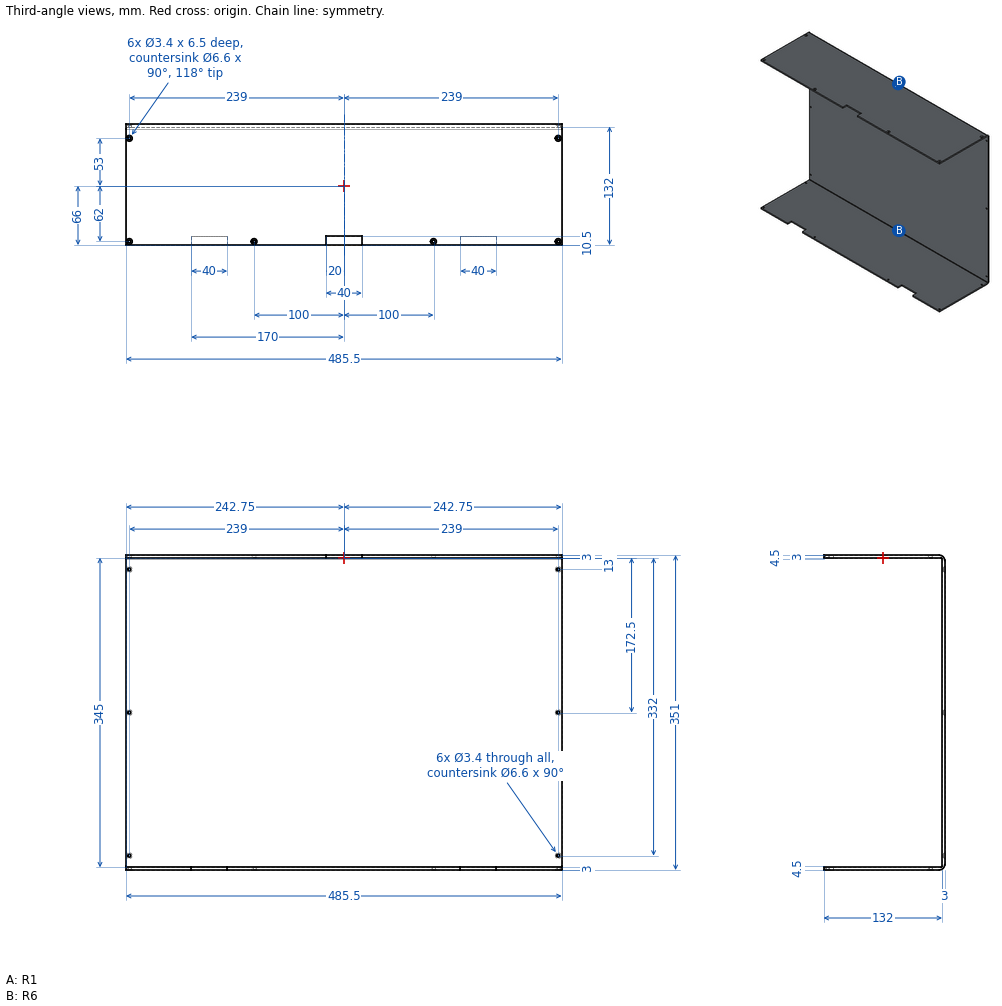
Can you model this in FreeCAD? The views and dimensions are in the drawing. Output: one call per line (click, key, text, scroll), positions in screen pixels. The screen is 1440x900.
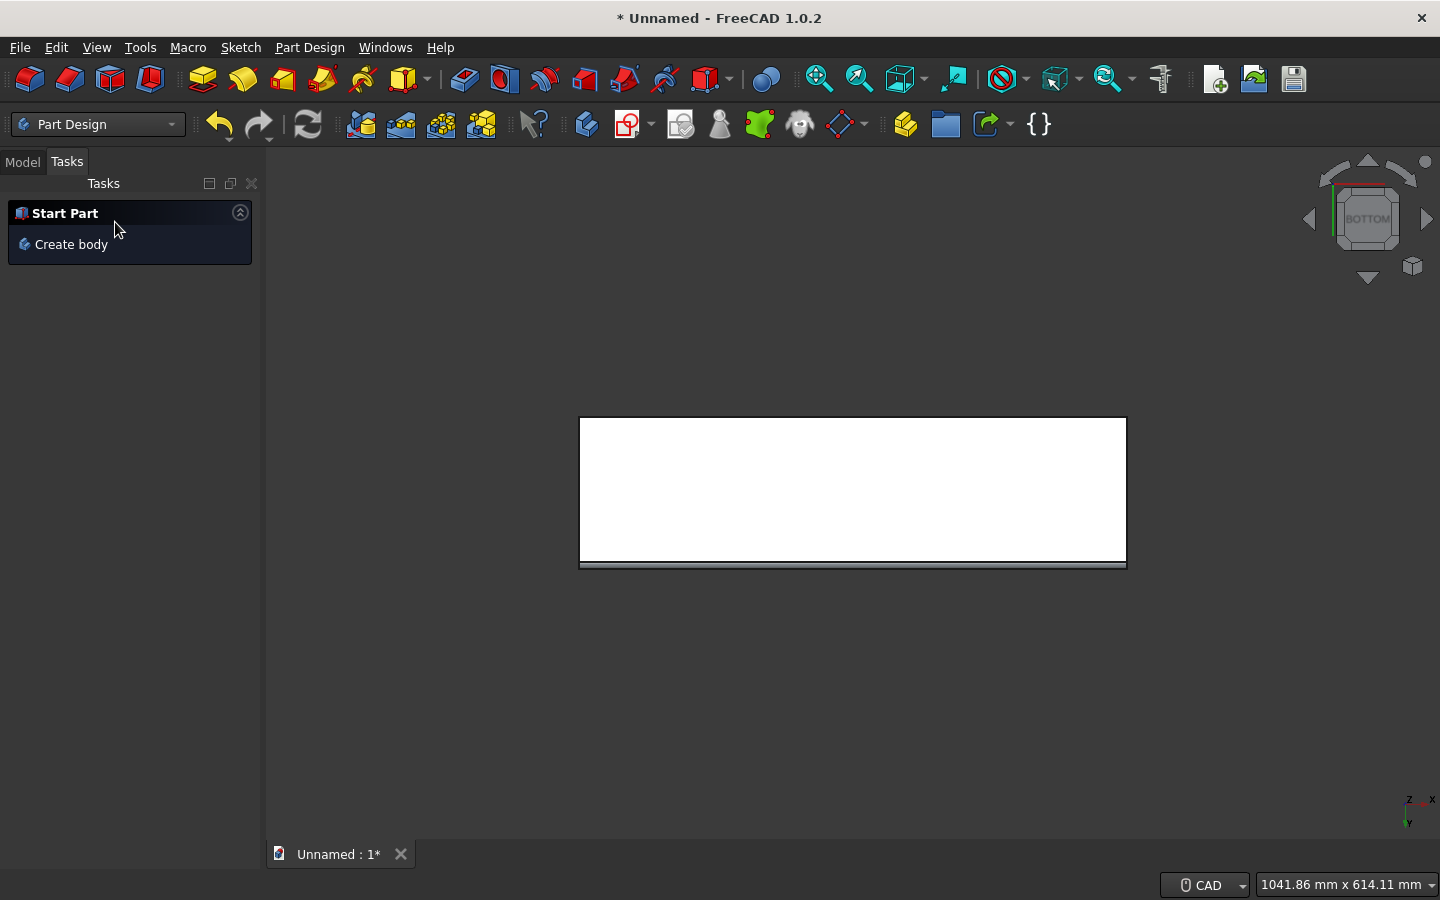
click(1009, 489)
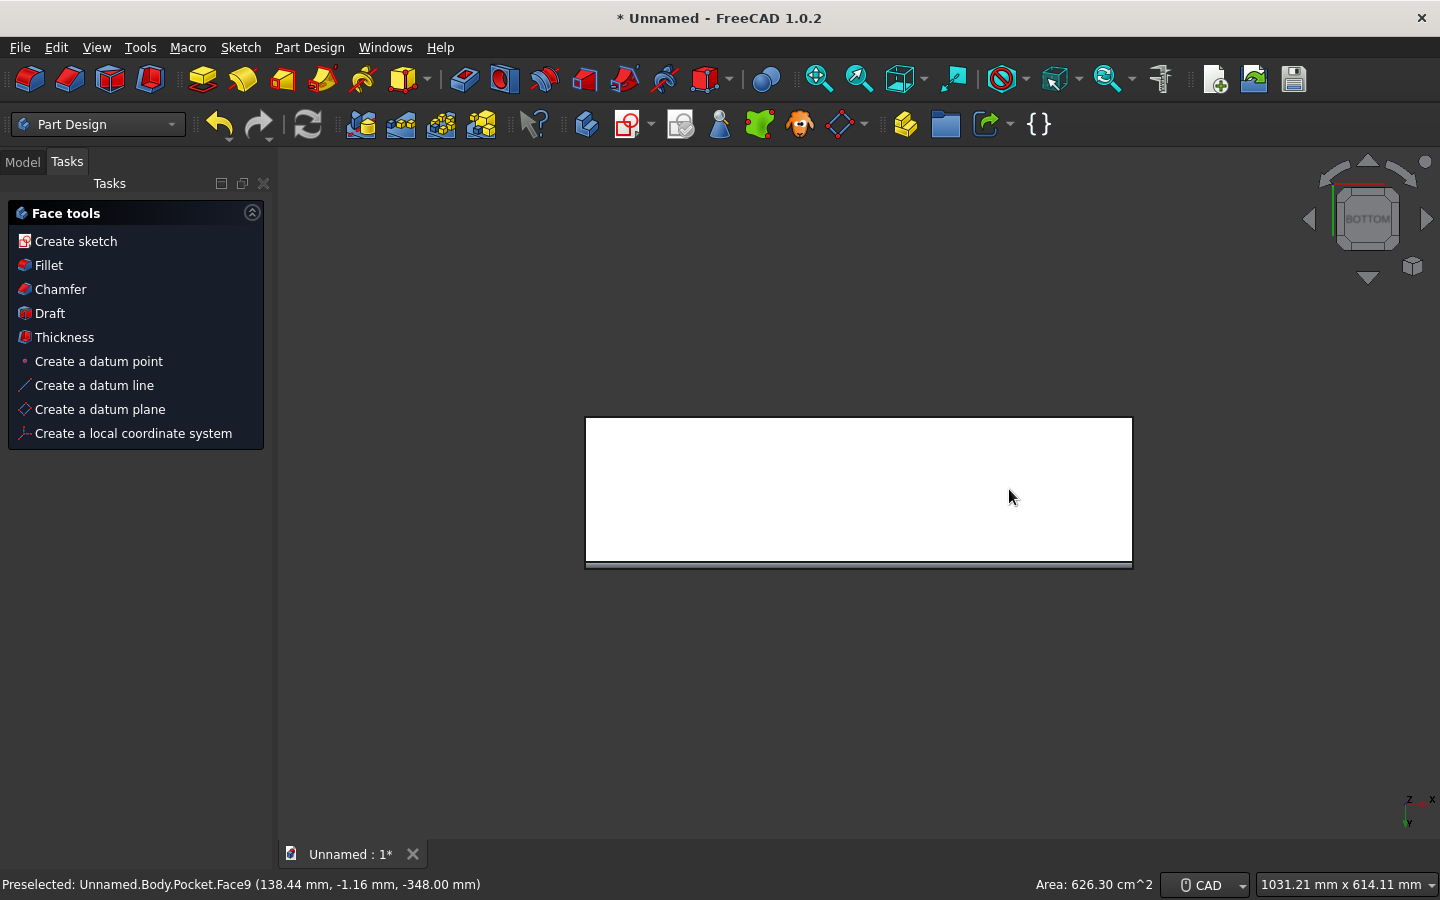
click(628, 124)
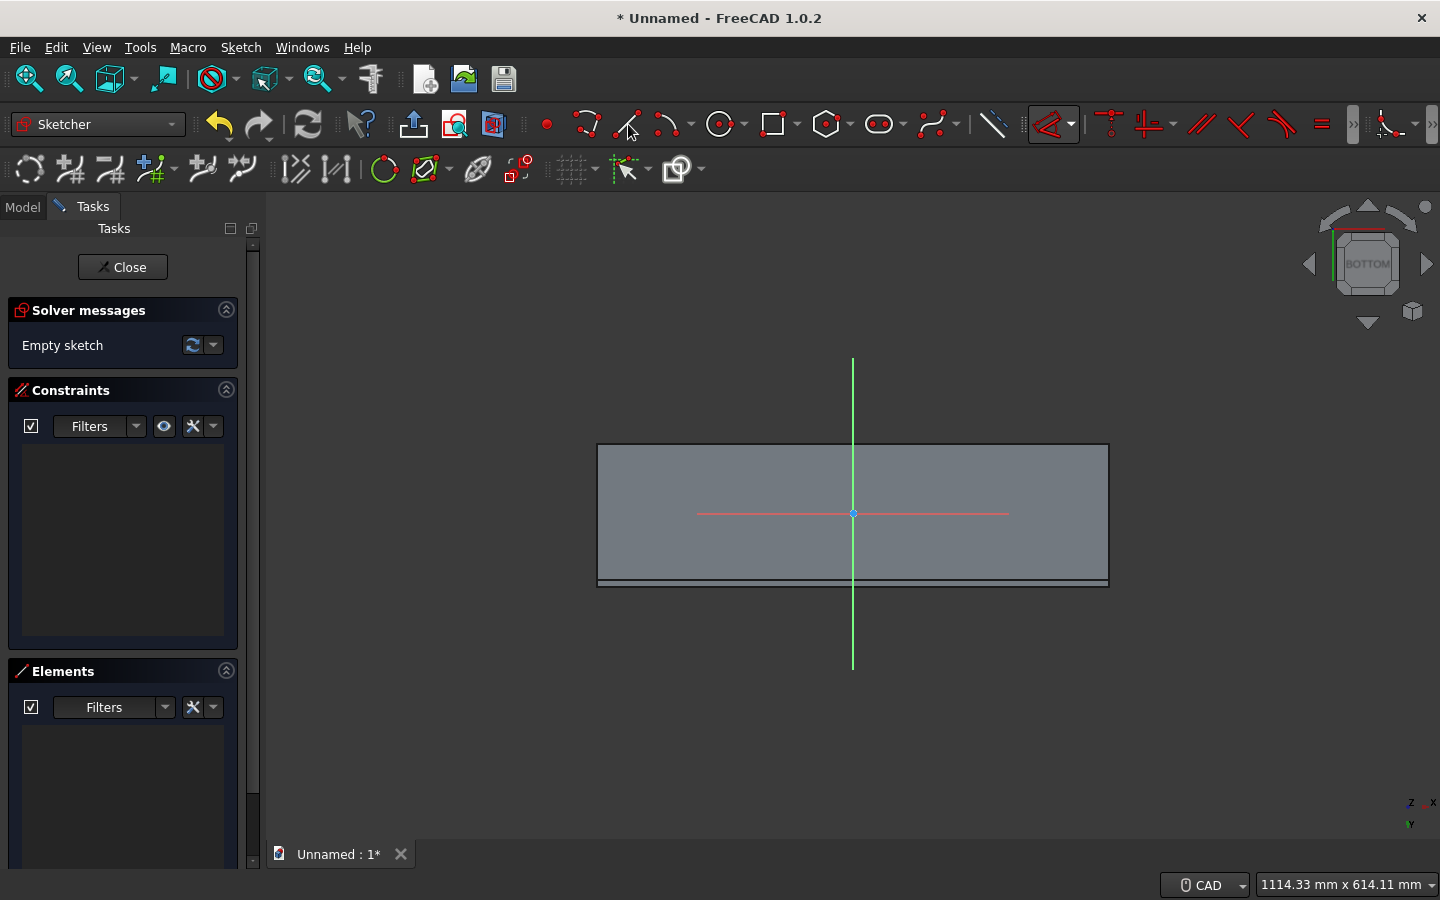
scroll(936, 435, up, 3)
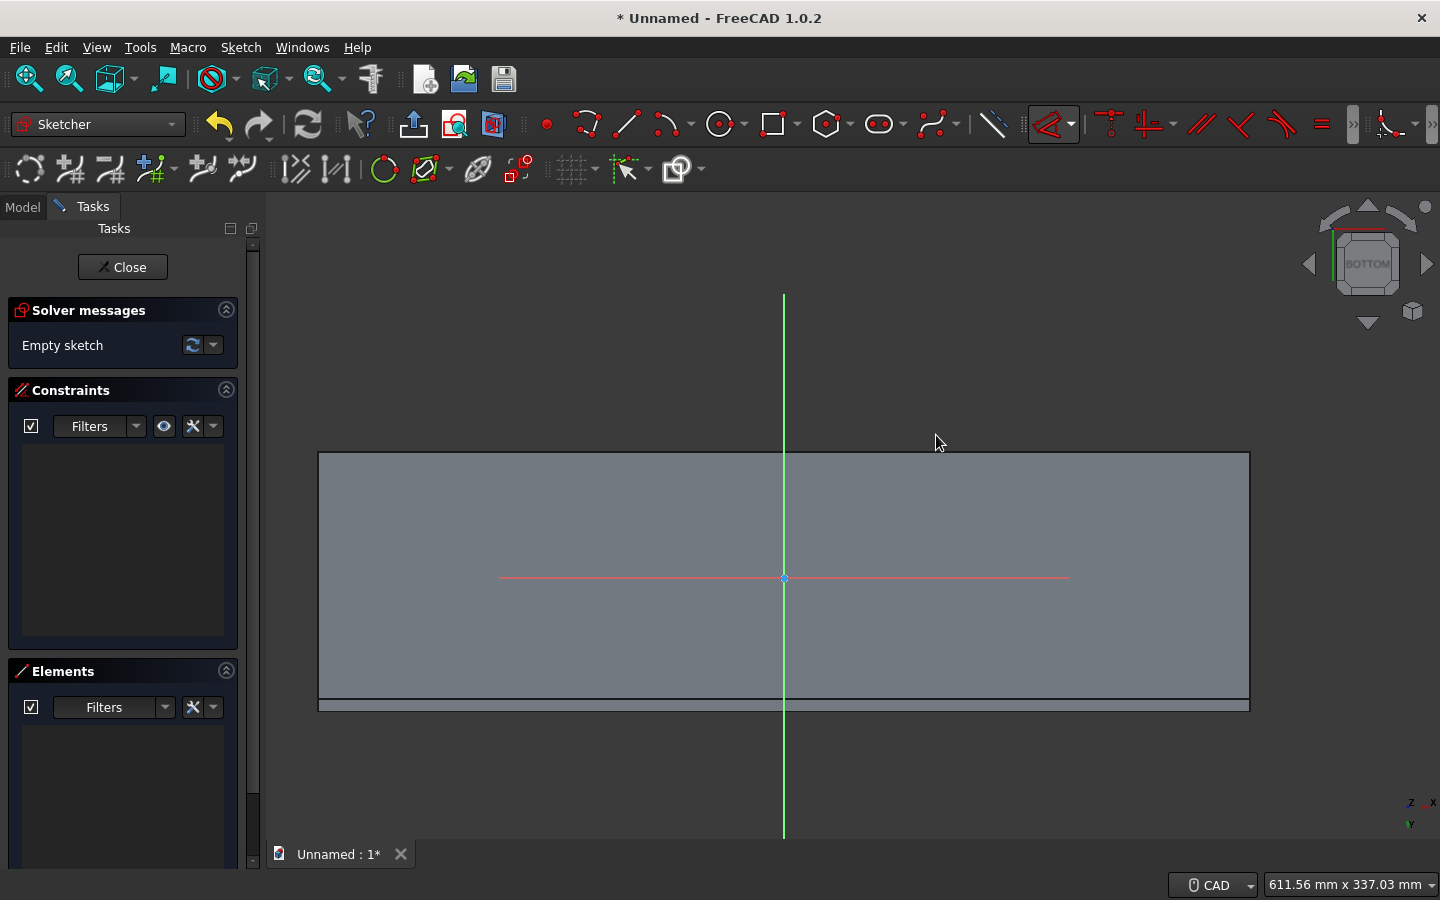
click(774, 124)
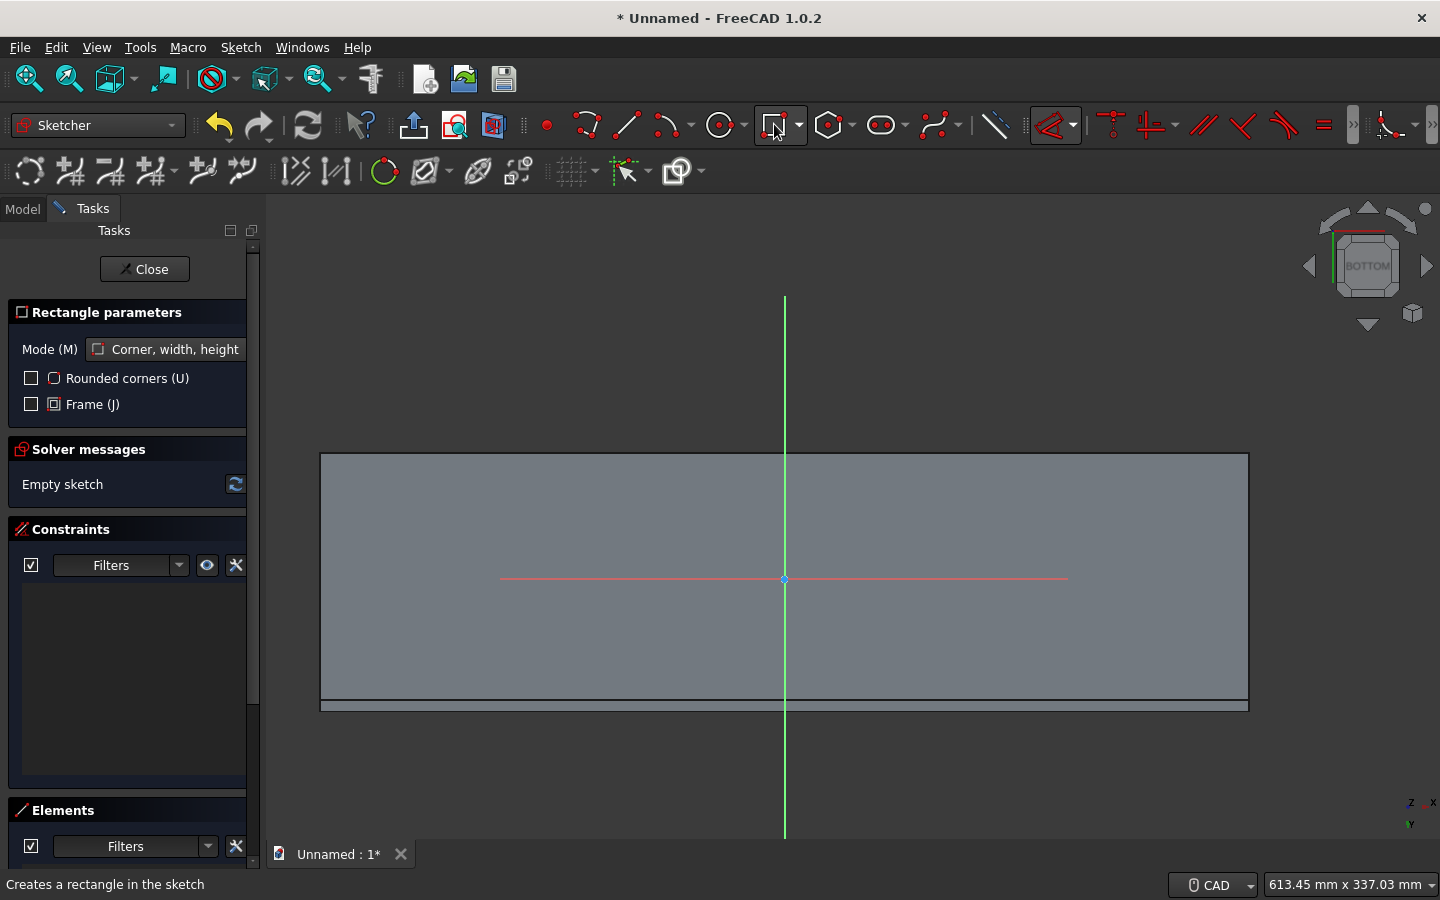
click(459, 453)
move(536, 473)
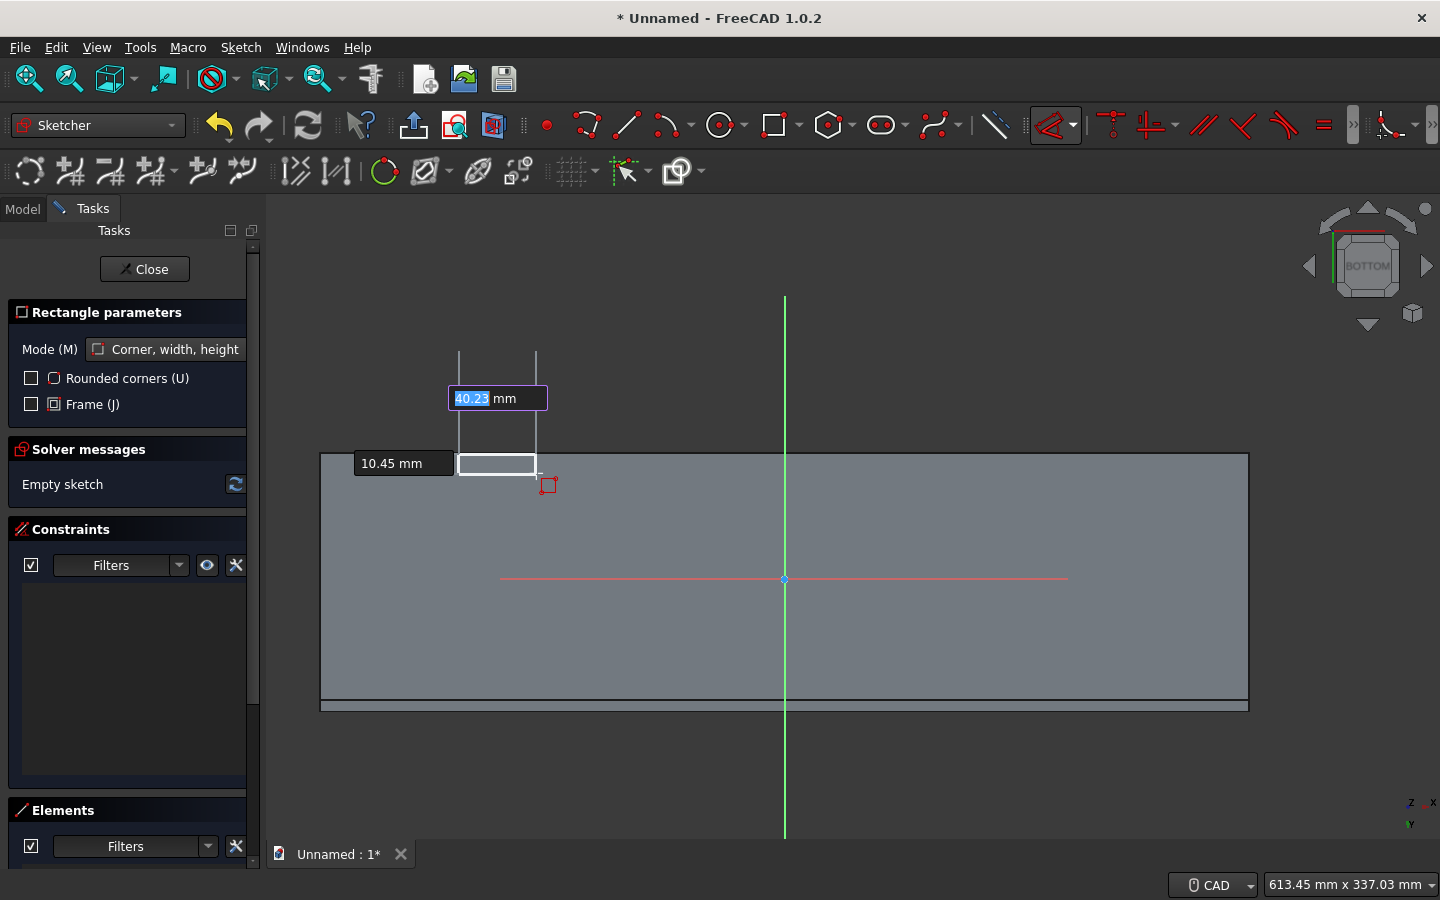
text(40)
key(Tab)
text(10.5)
key(Return)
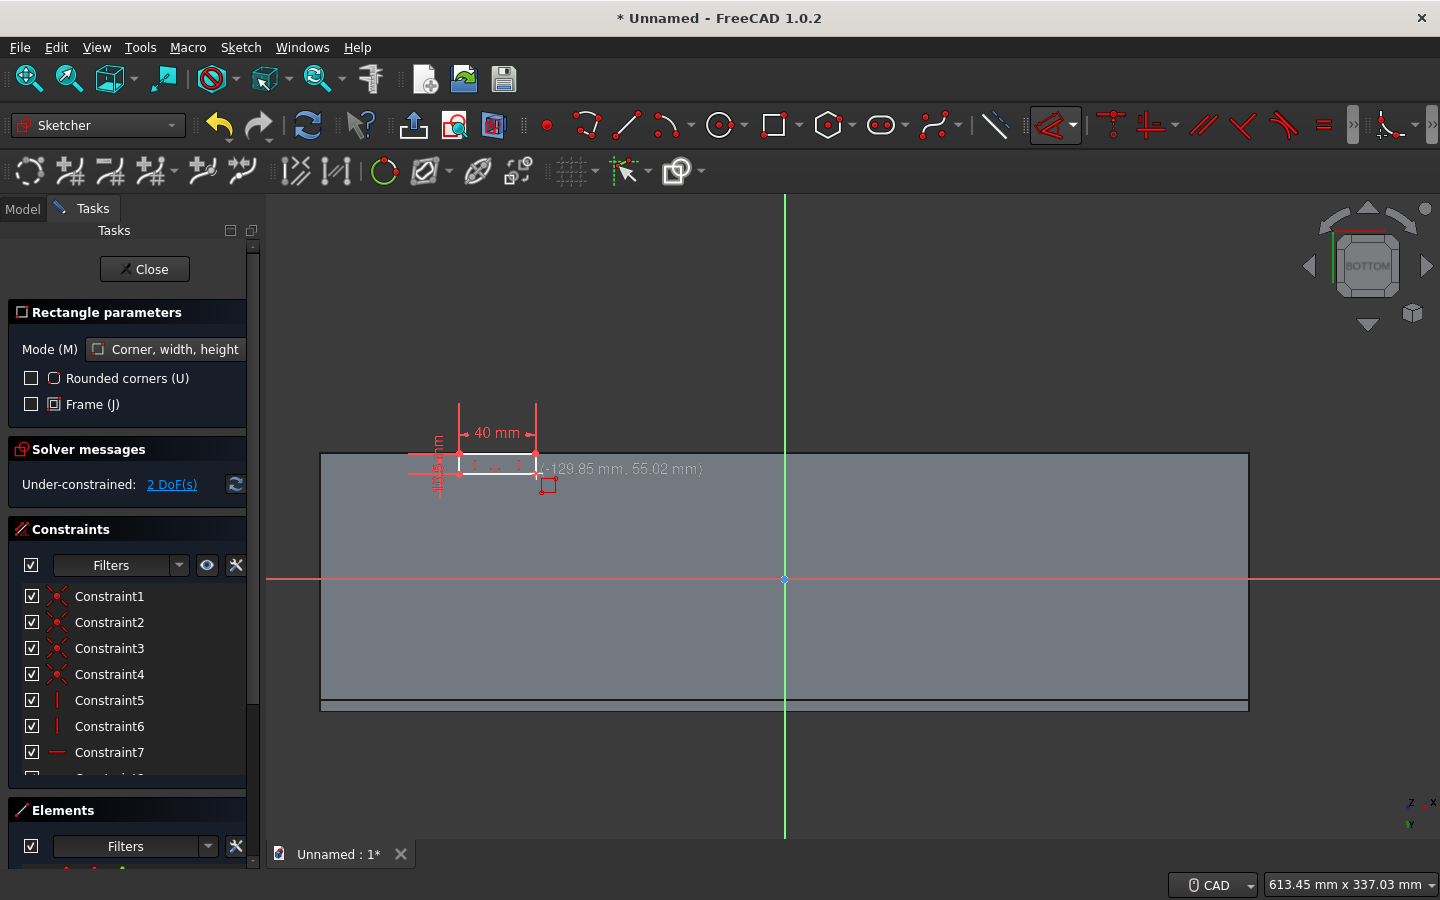
click(1033, 453)
move(1110, 473)